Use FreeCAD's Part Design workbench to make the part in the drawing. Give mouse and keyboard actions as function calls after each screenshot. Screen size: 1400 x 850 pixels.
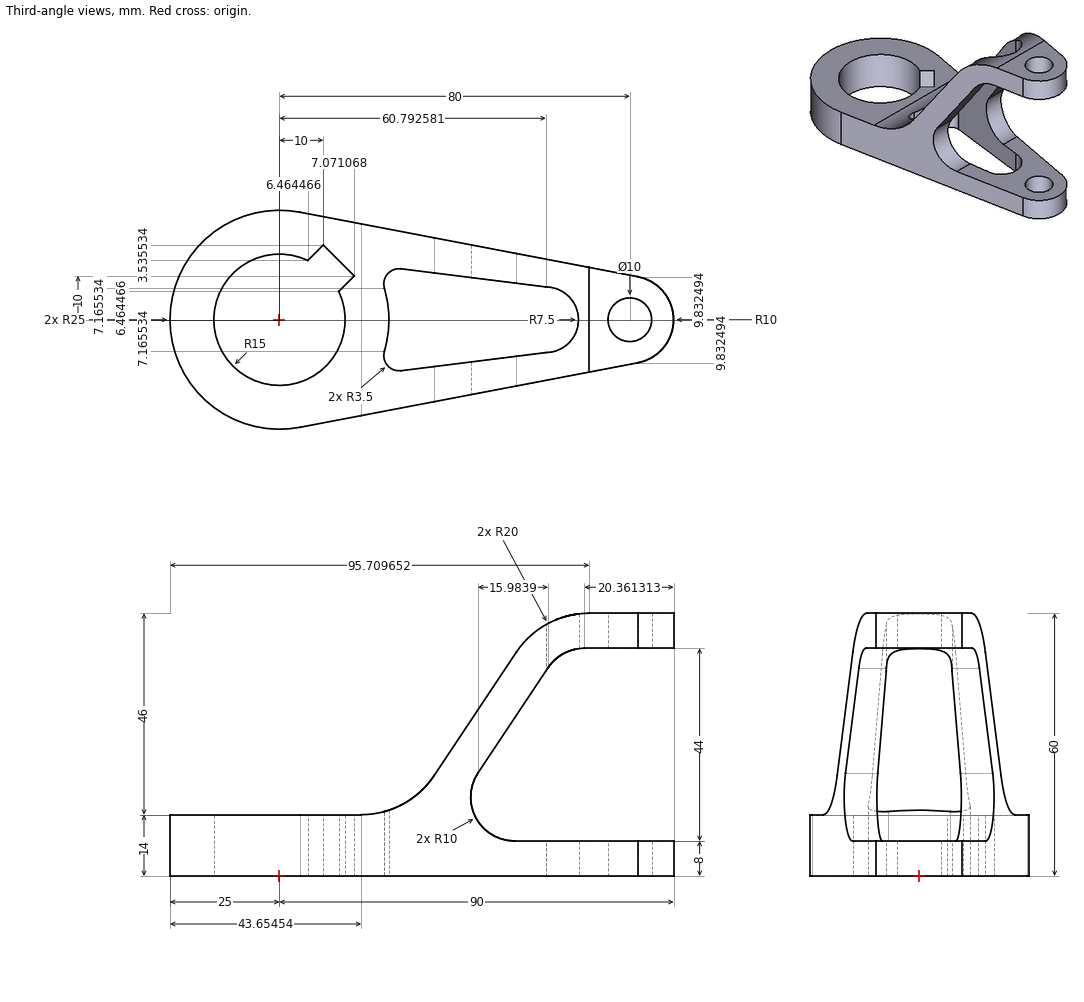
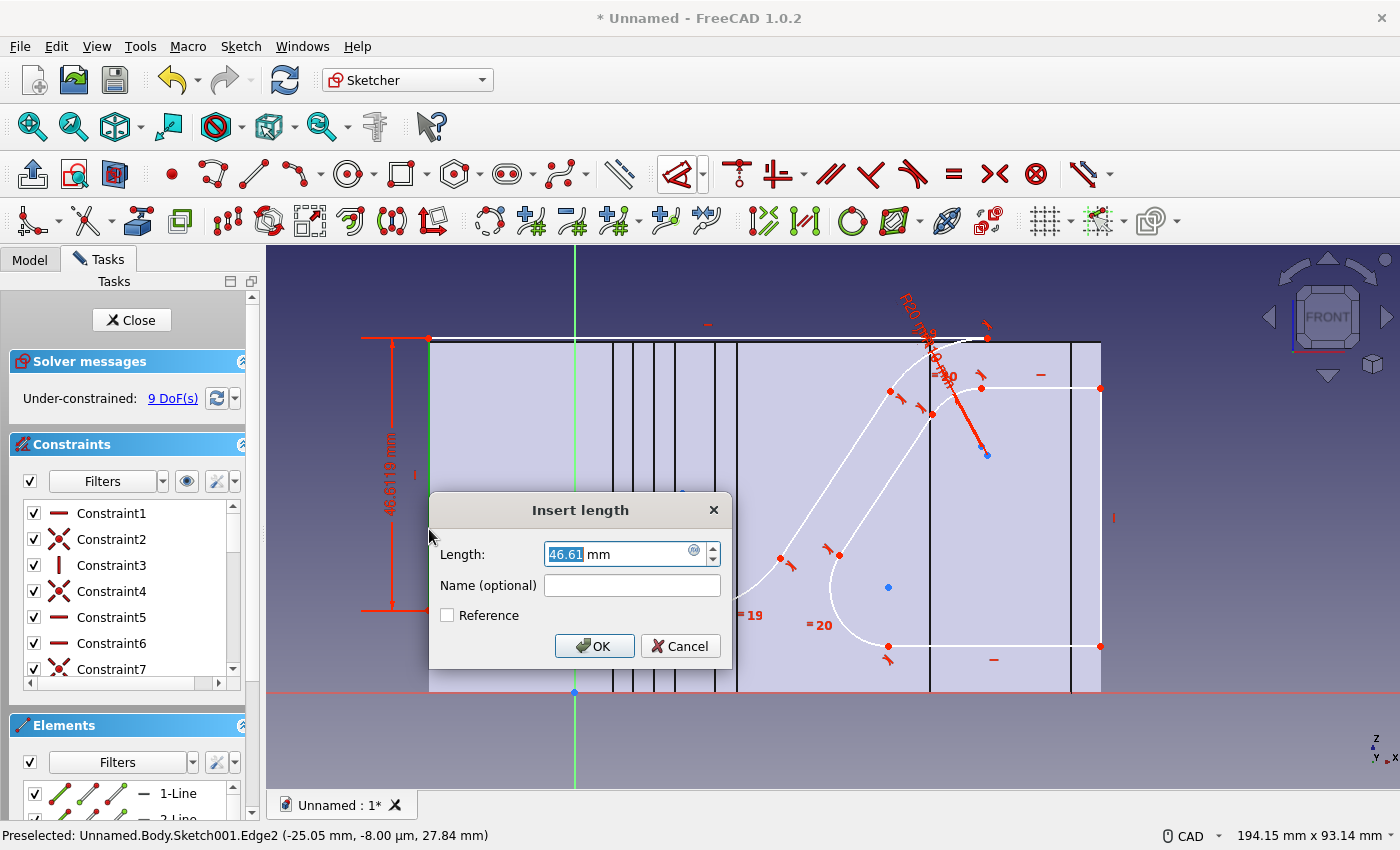
text(46)
key(Return)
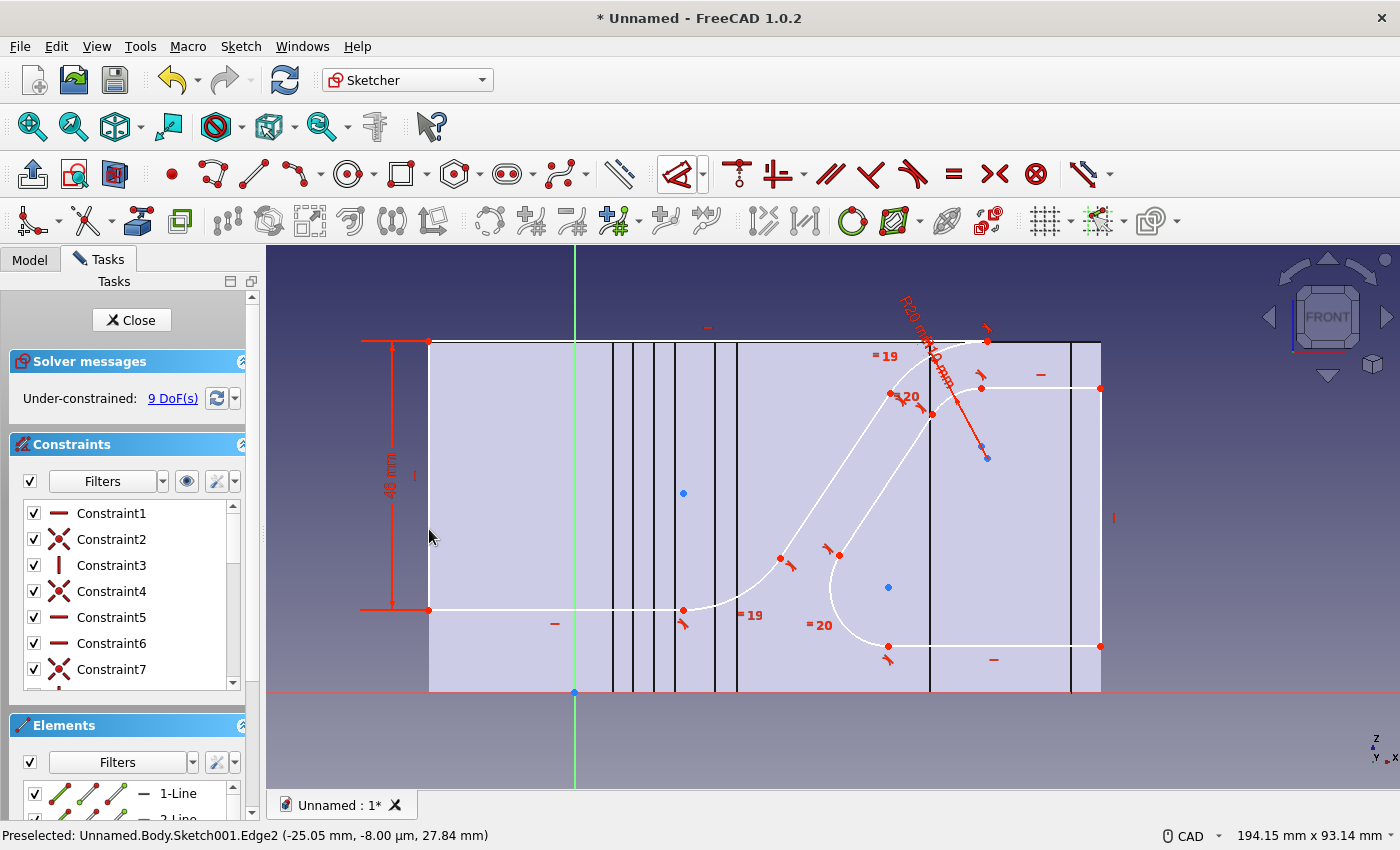
click(1101, 466)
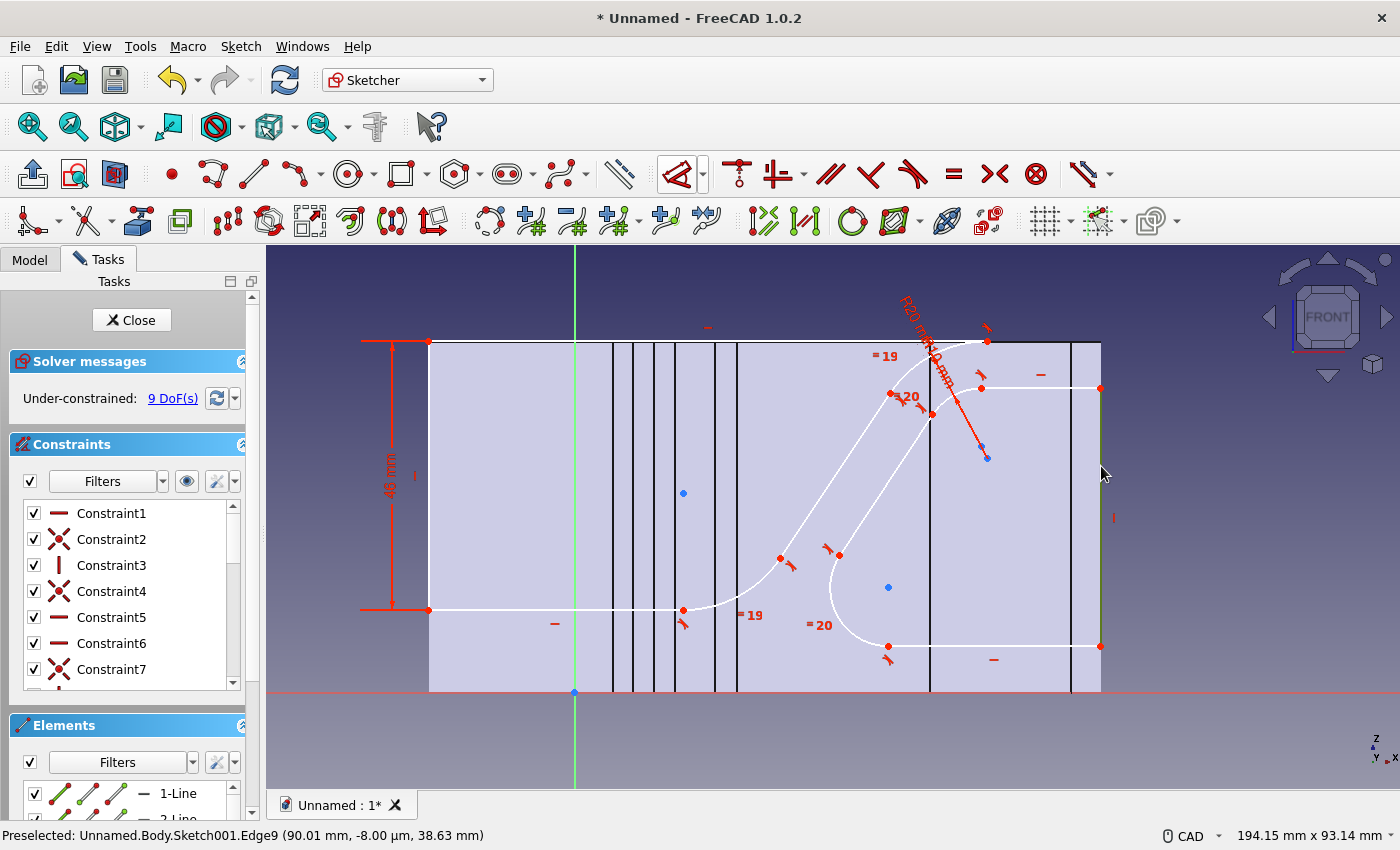
click(702, 174)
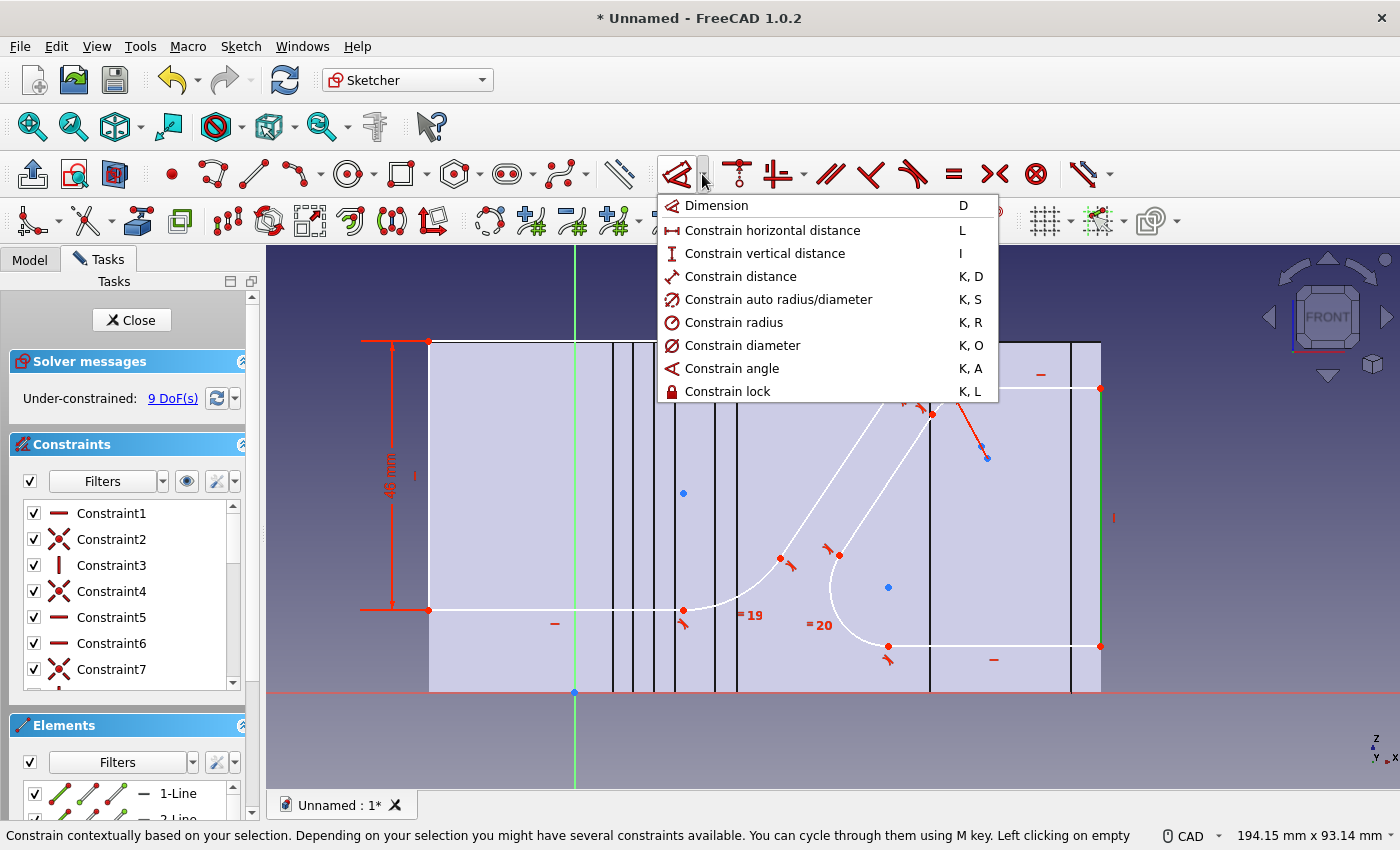
click(828, 254)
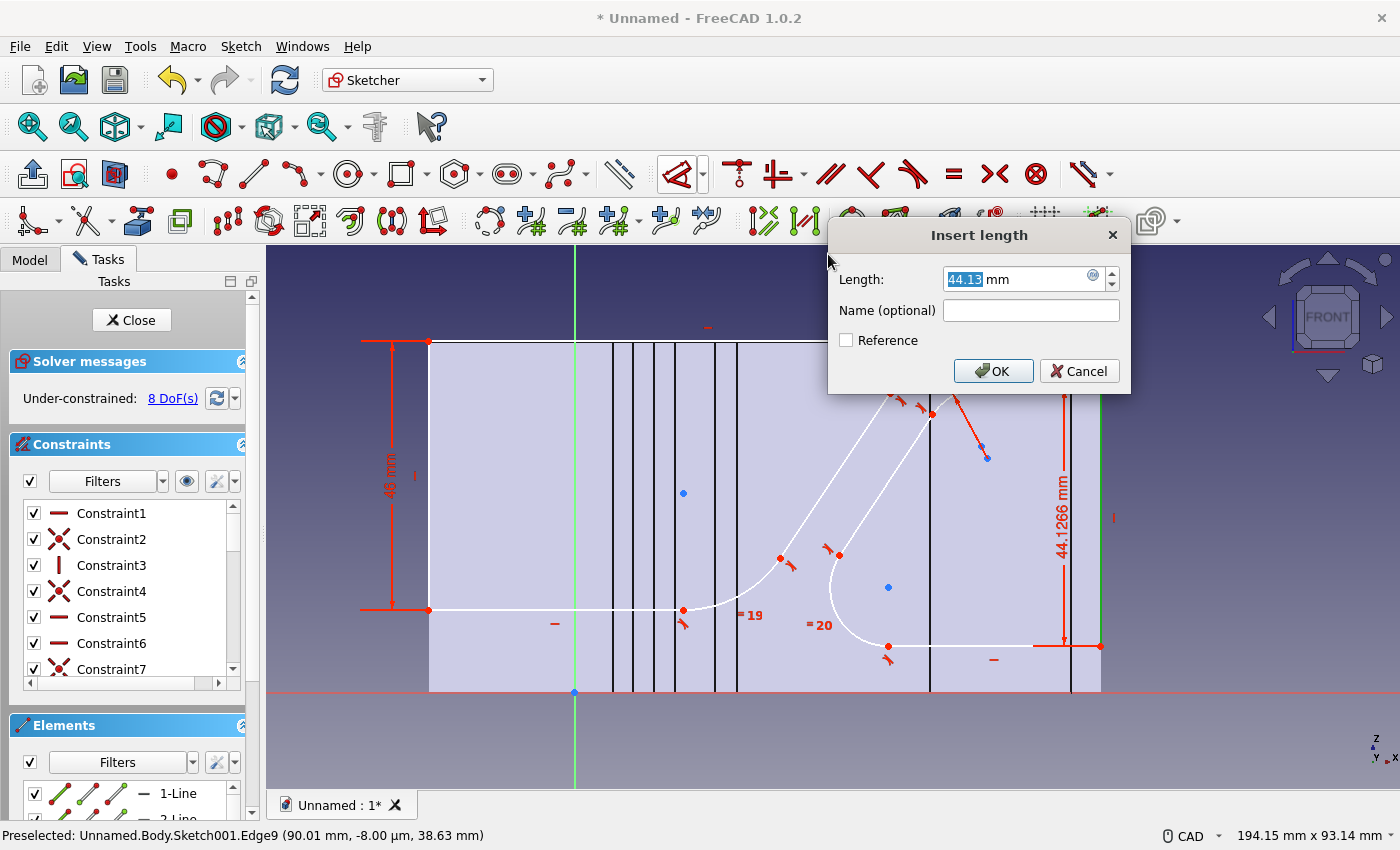
text(44)
key(Return)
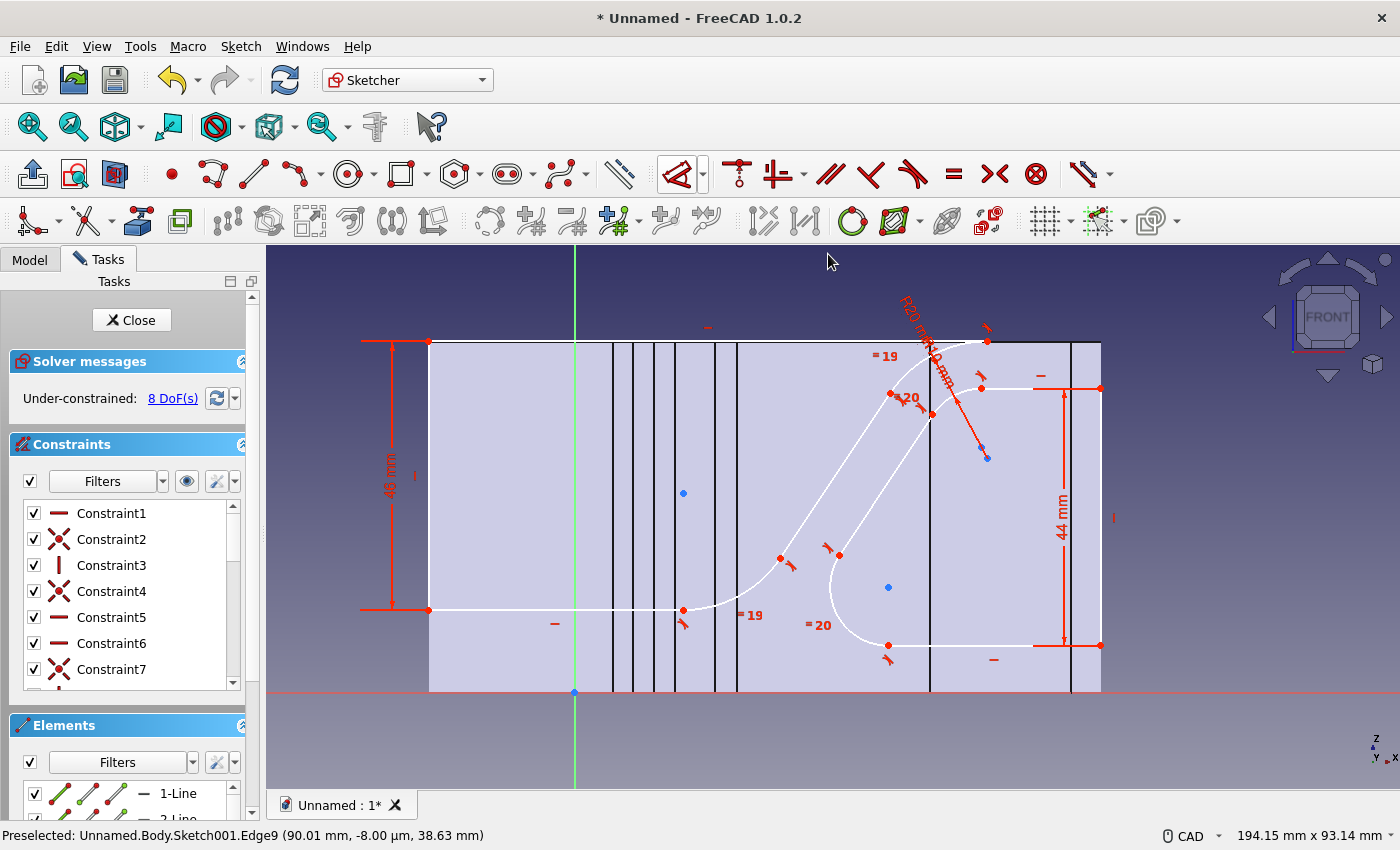
click(1101, 646)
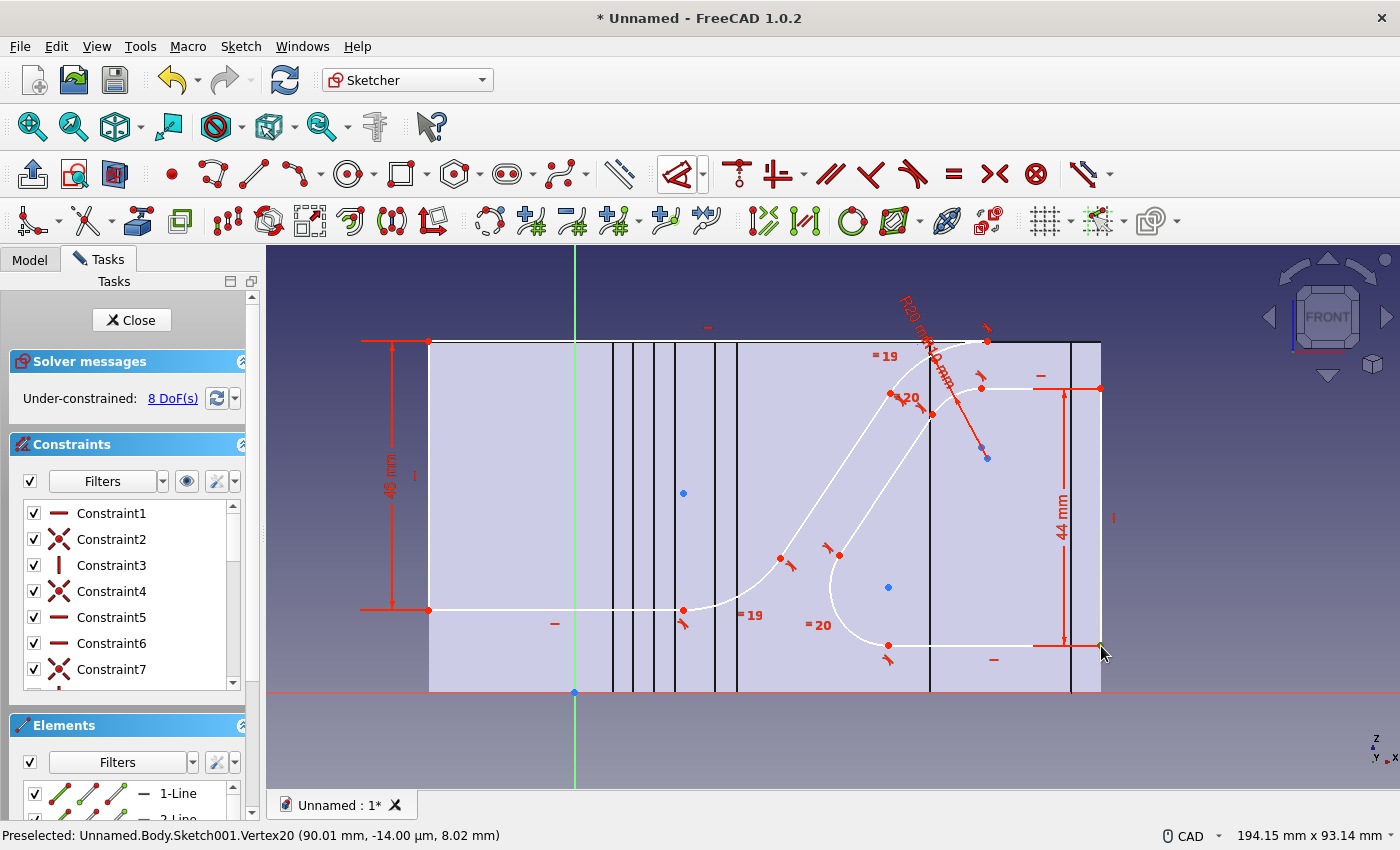
key(i)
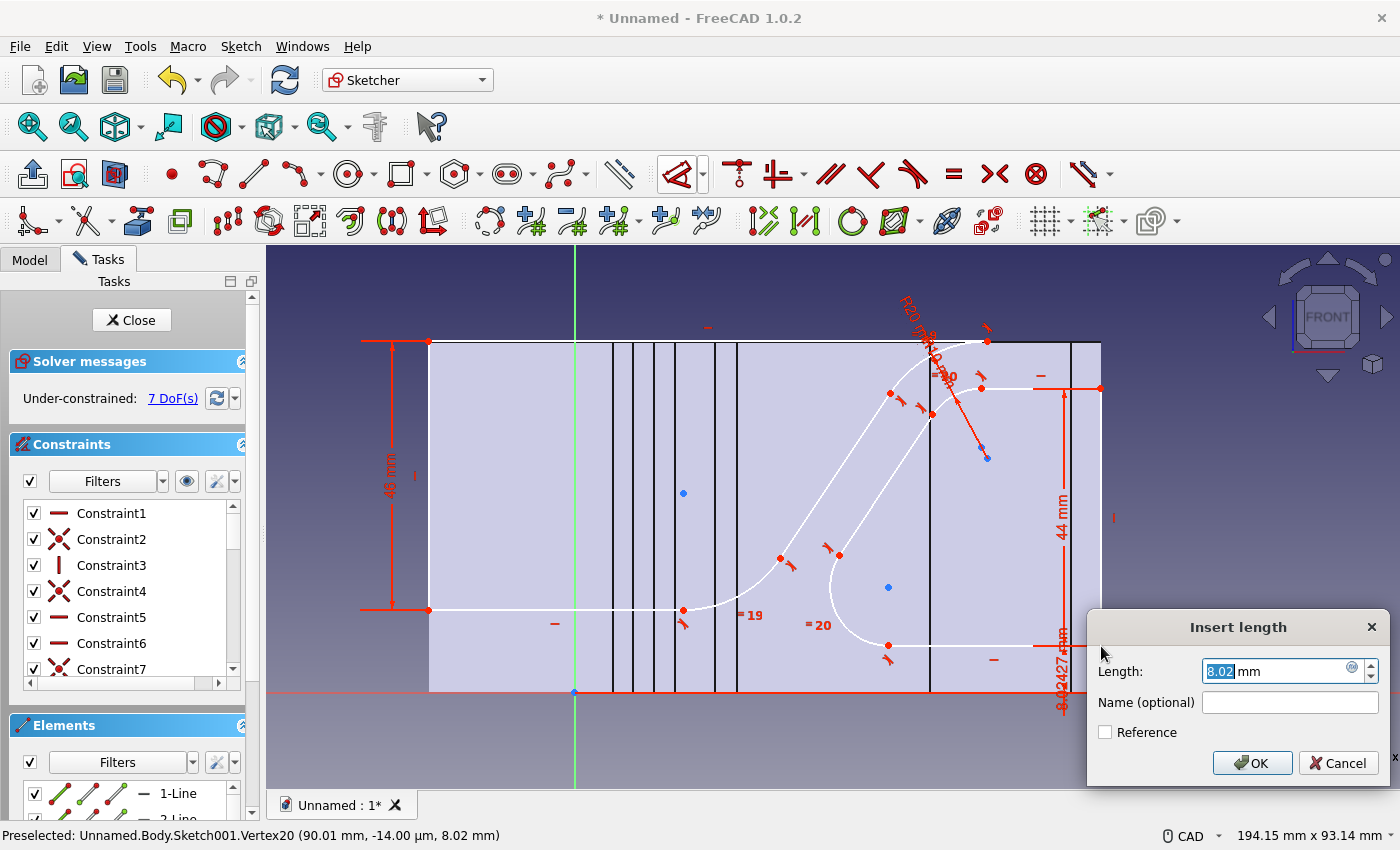
text(8)
key(Return)